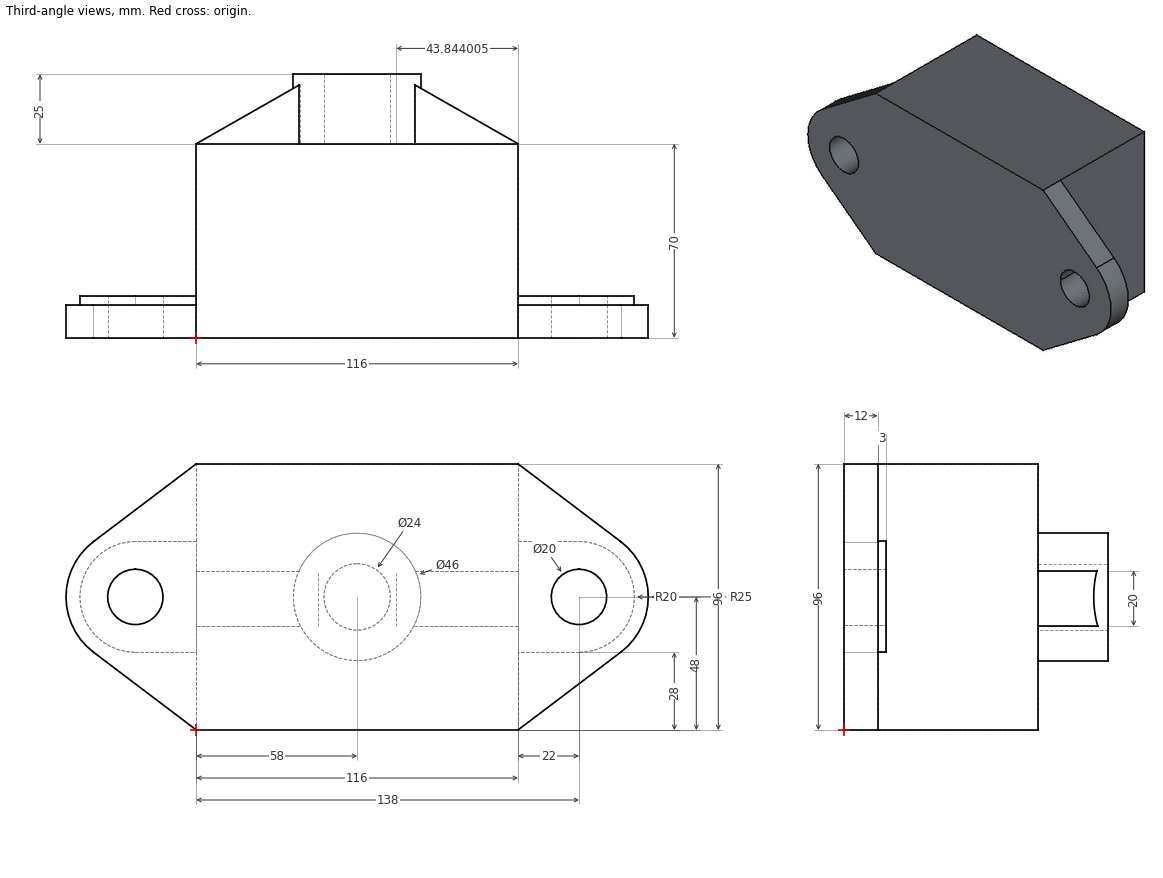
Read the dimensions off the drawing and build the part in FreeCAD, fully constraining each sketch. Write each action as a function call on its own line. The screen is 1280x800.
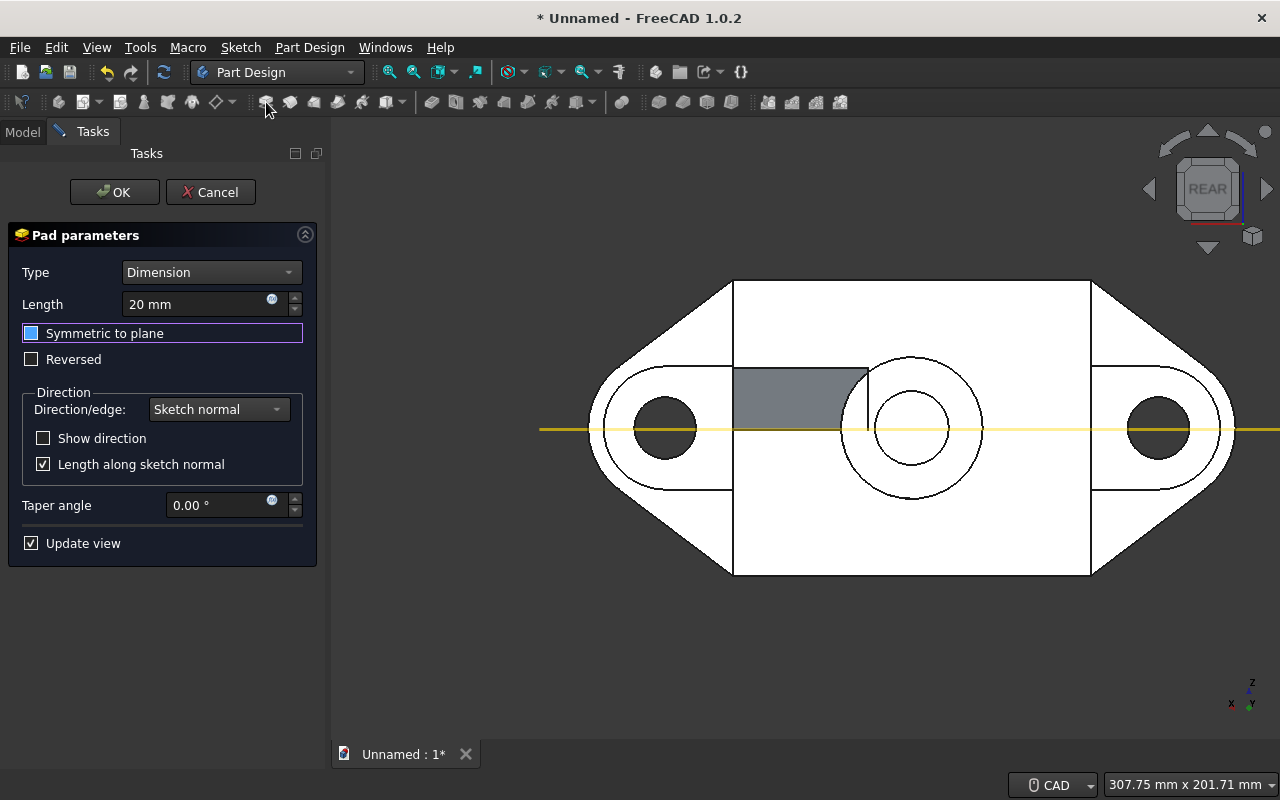
click(30, 333)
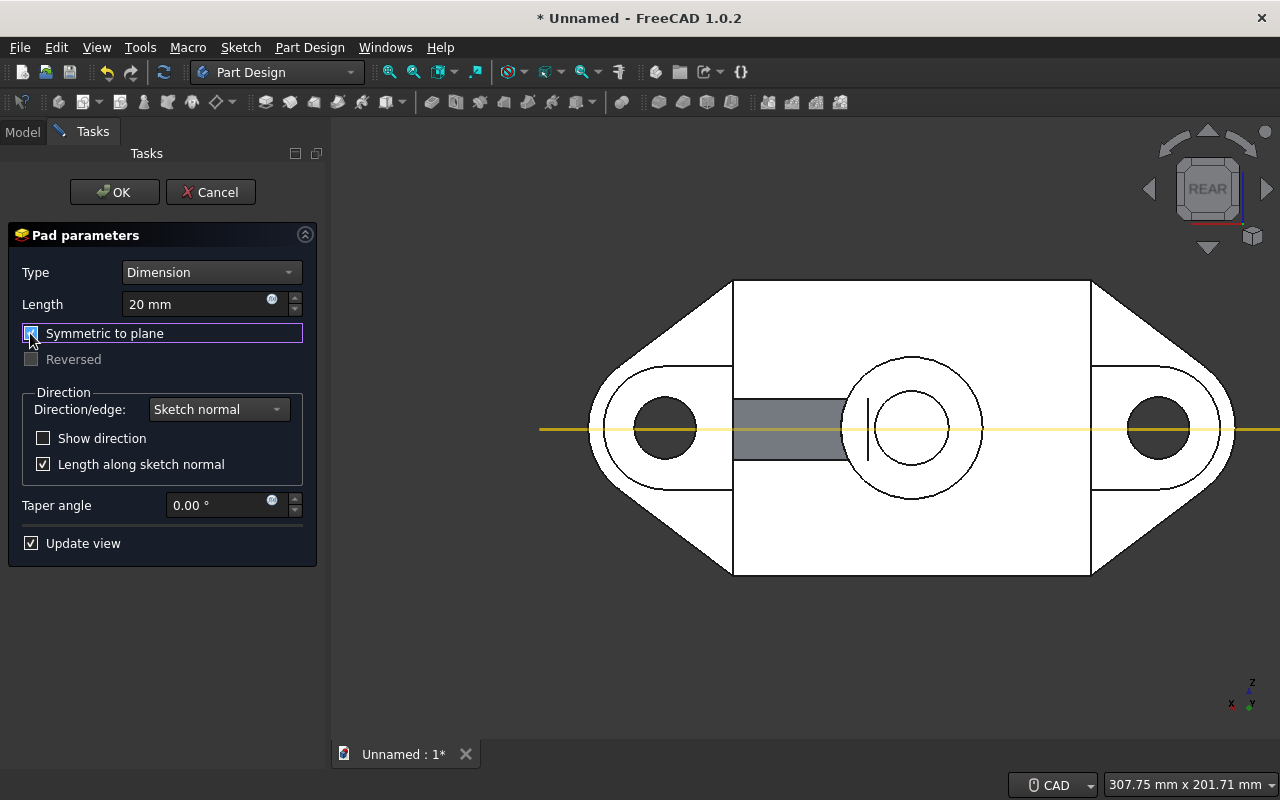
click(115, 192)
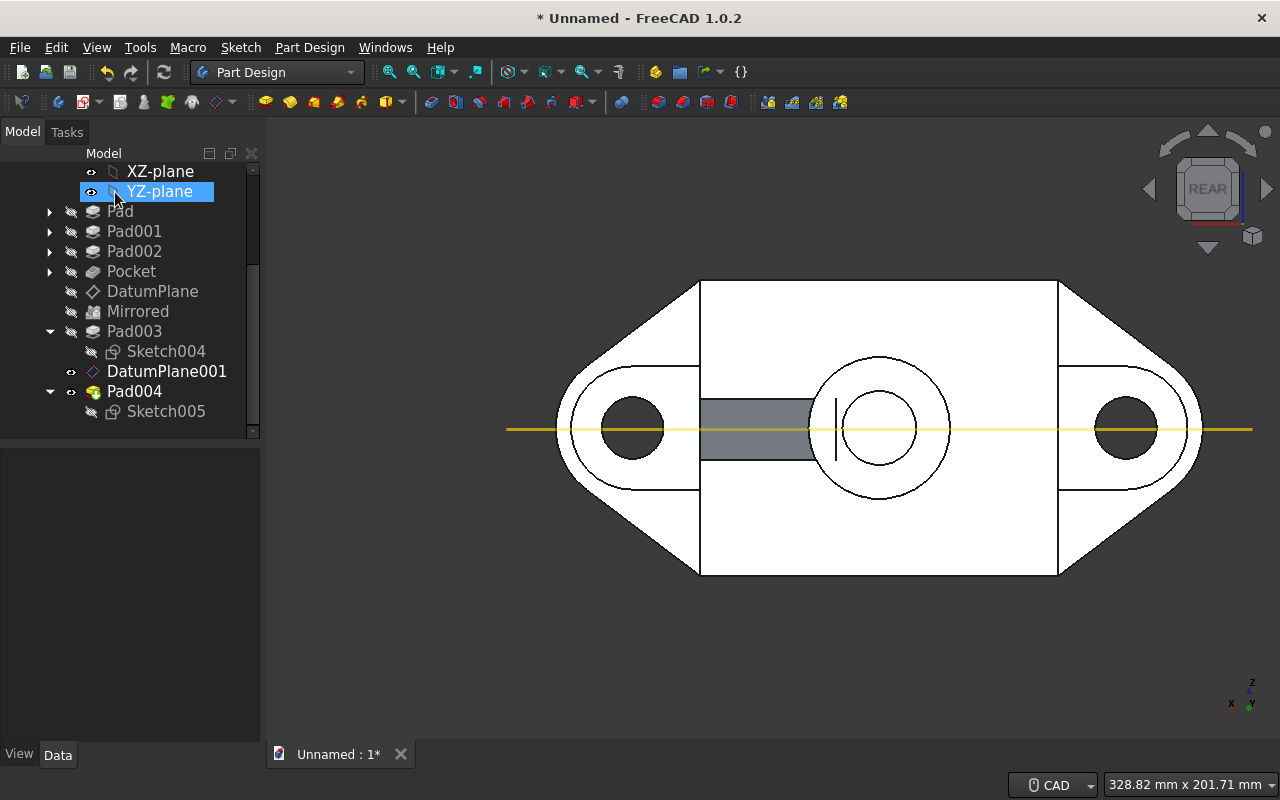
click(116, 372)
key(space)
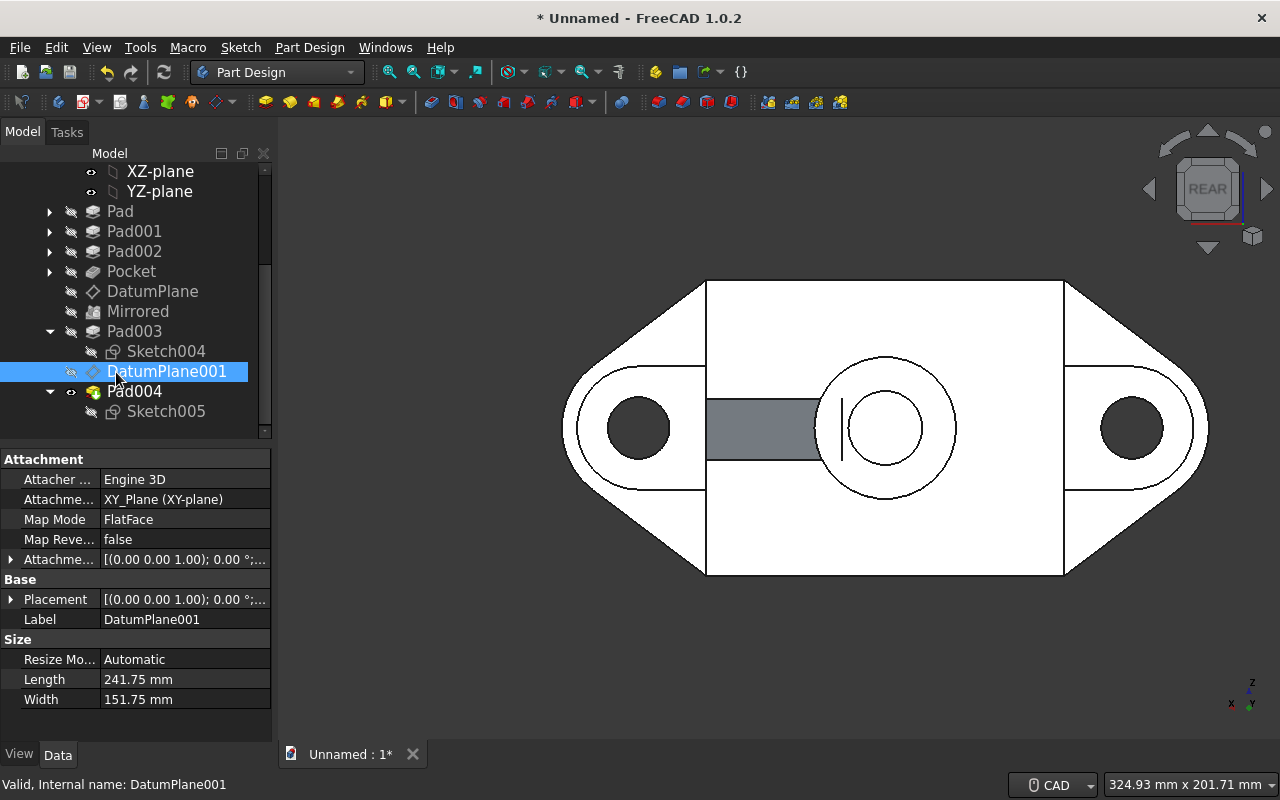
scroll(160, 287, down, 3)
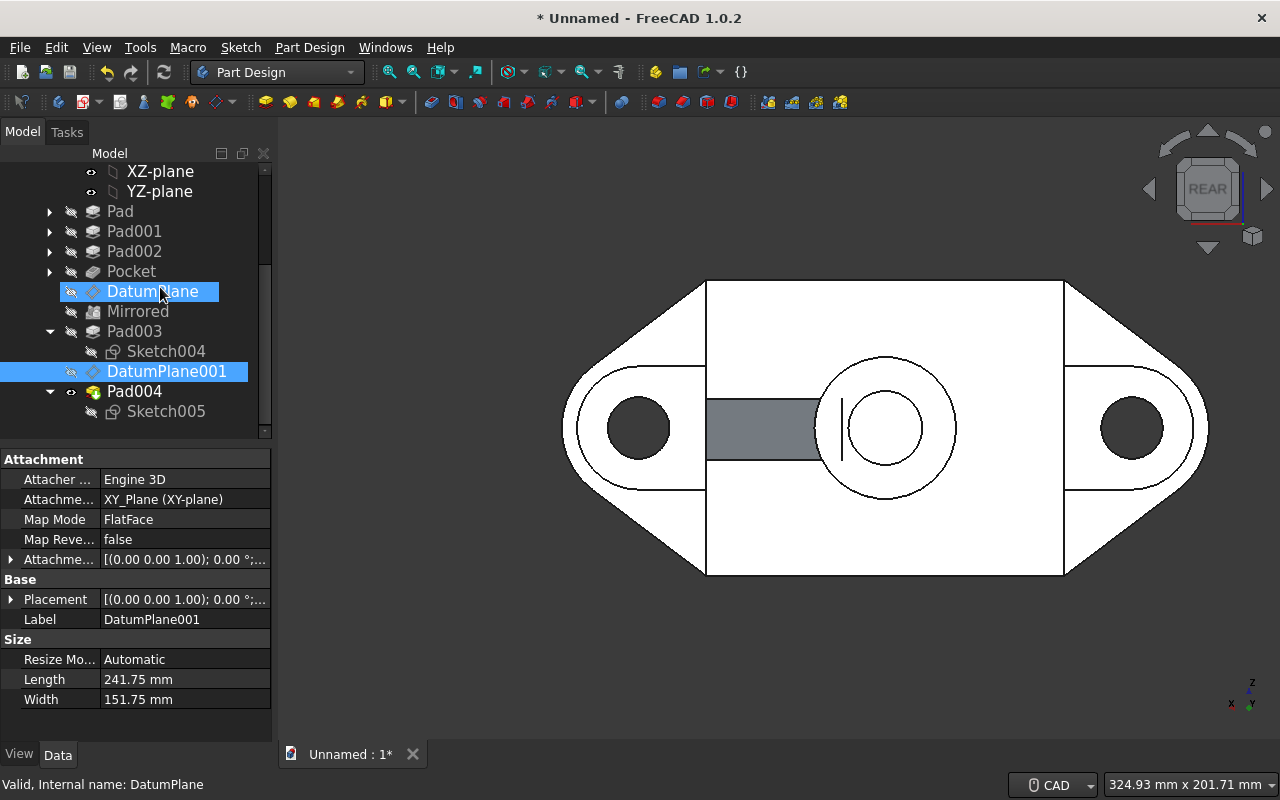
scroll(160, 287, up, 15)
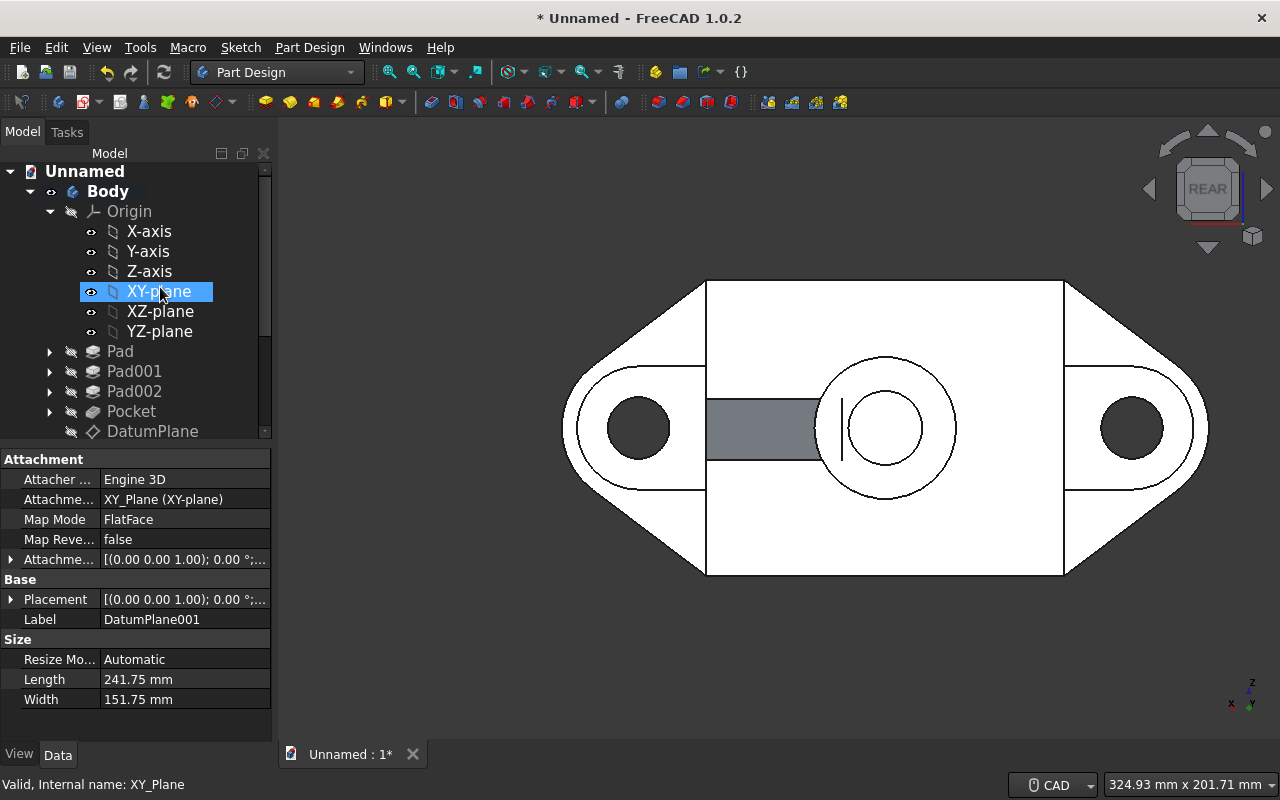
click(136, 332)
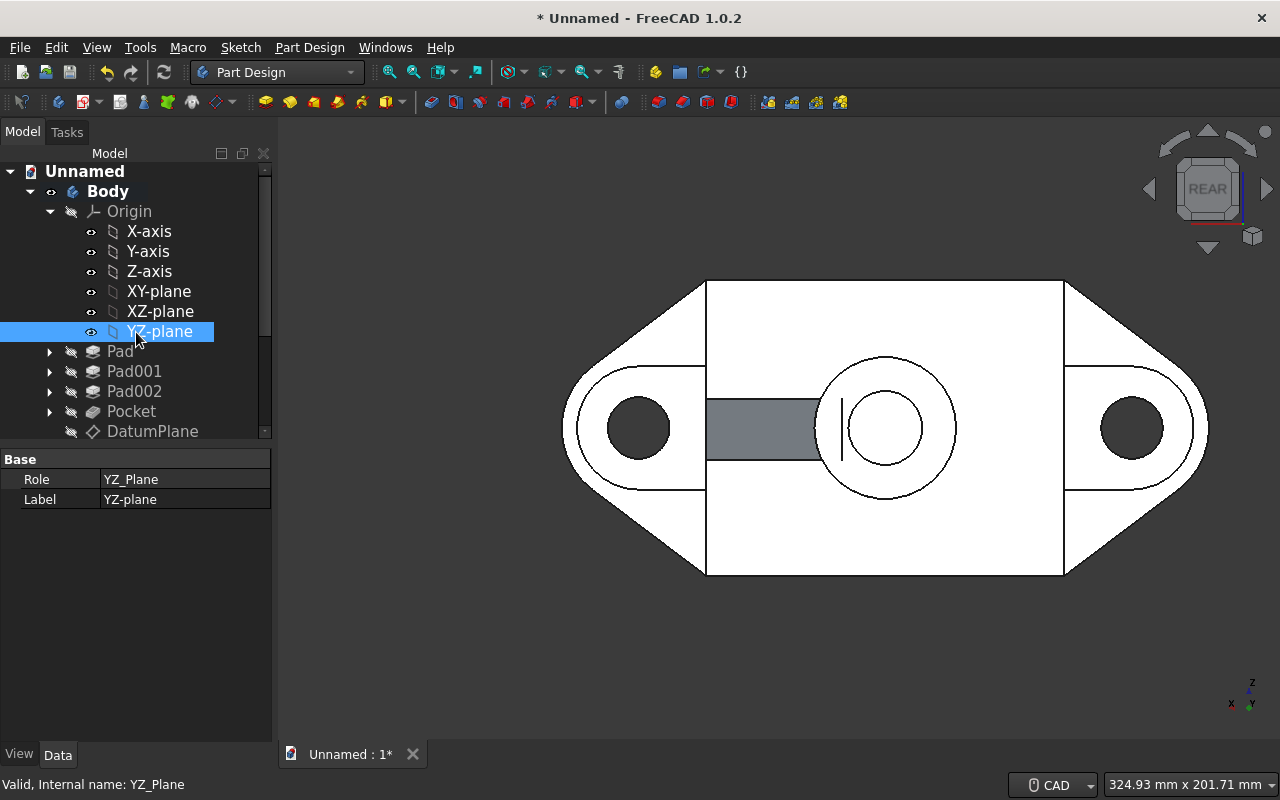
click(216, 102)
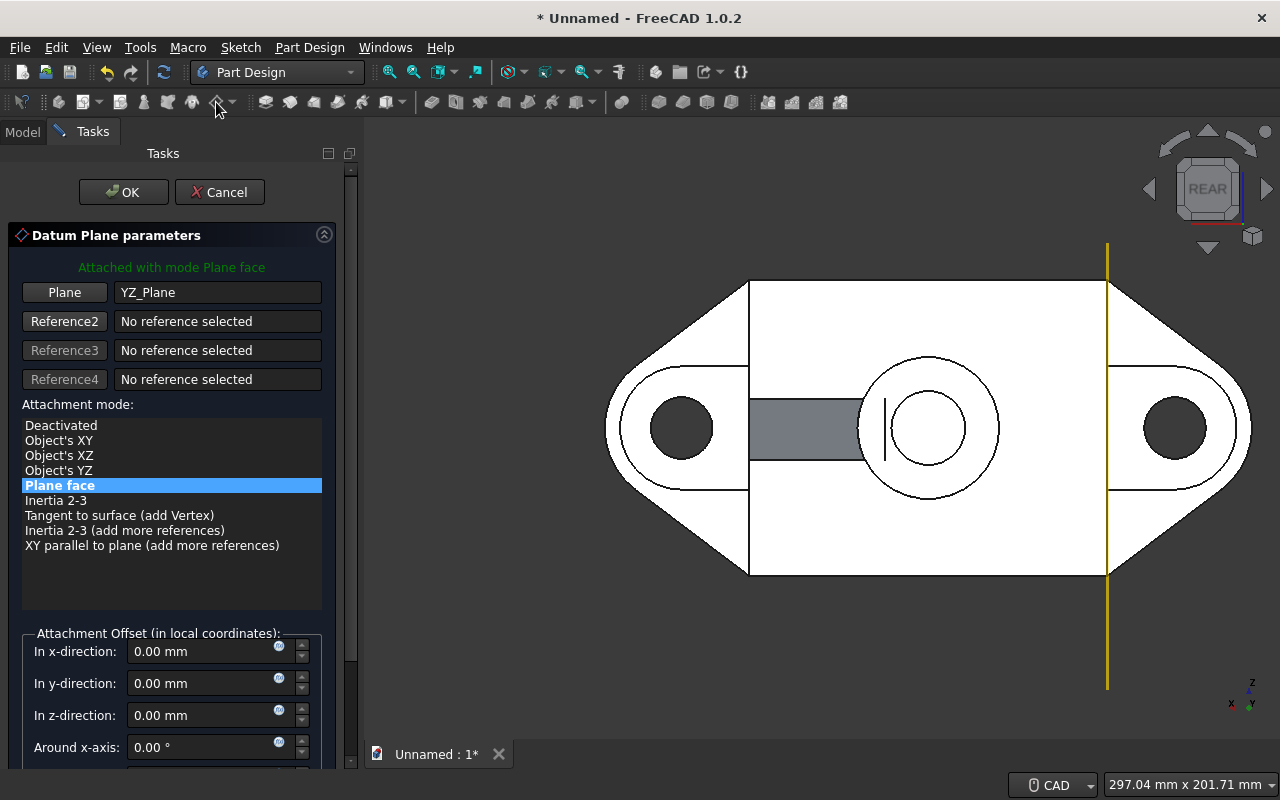
triple_click(210, 715)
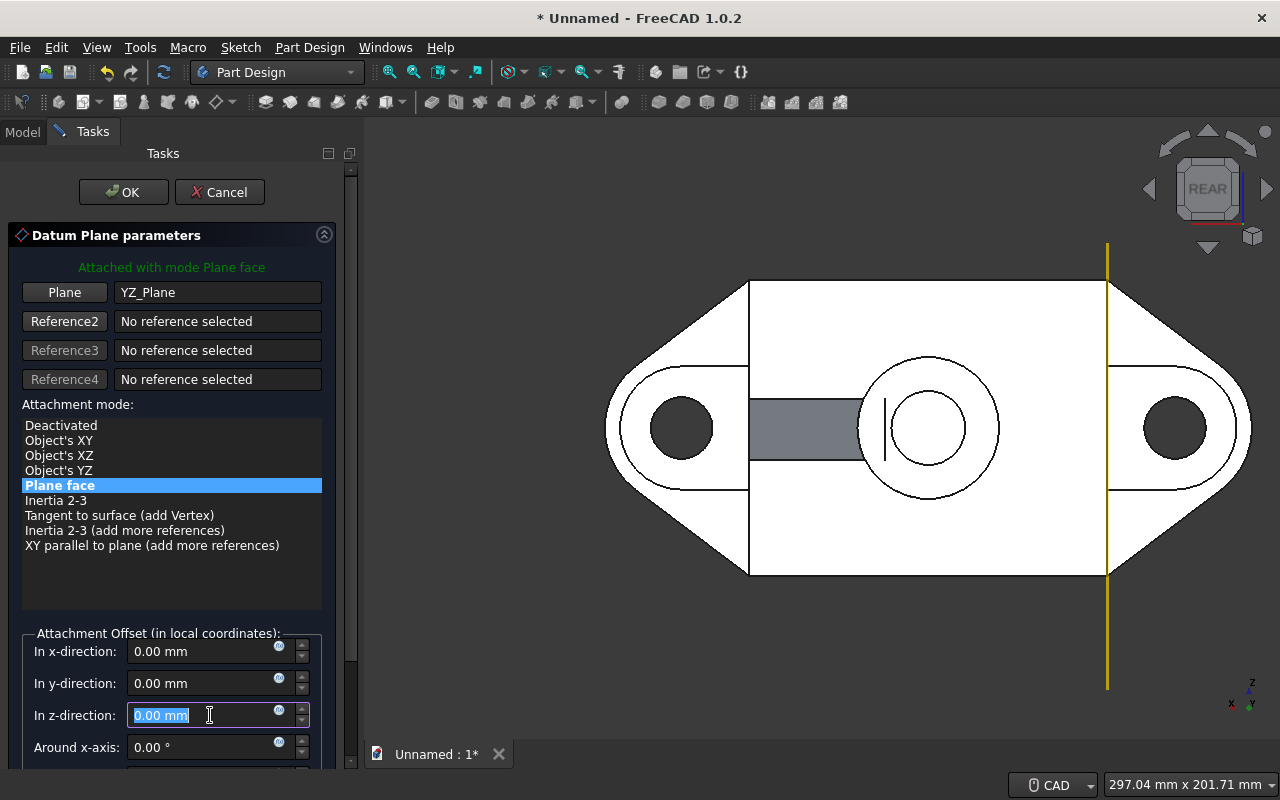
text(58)
key(Tab)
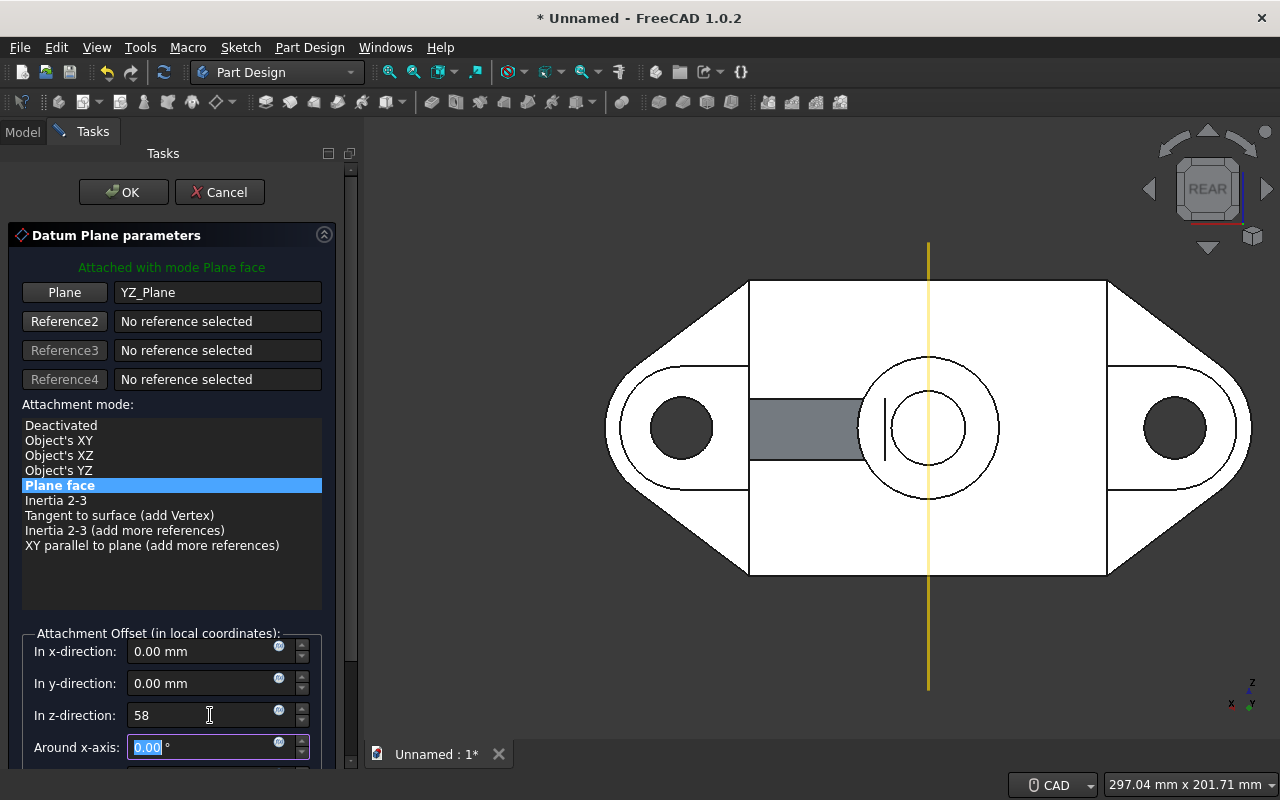
click(124, 192)